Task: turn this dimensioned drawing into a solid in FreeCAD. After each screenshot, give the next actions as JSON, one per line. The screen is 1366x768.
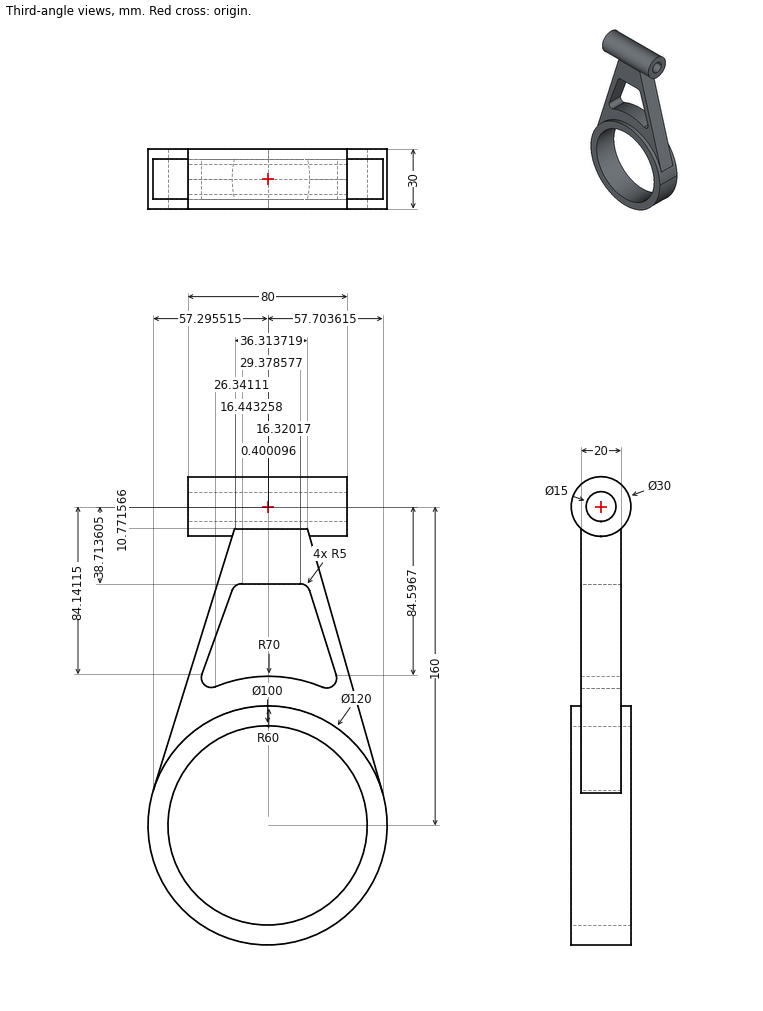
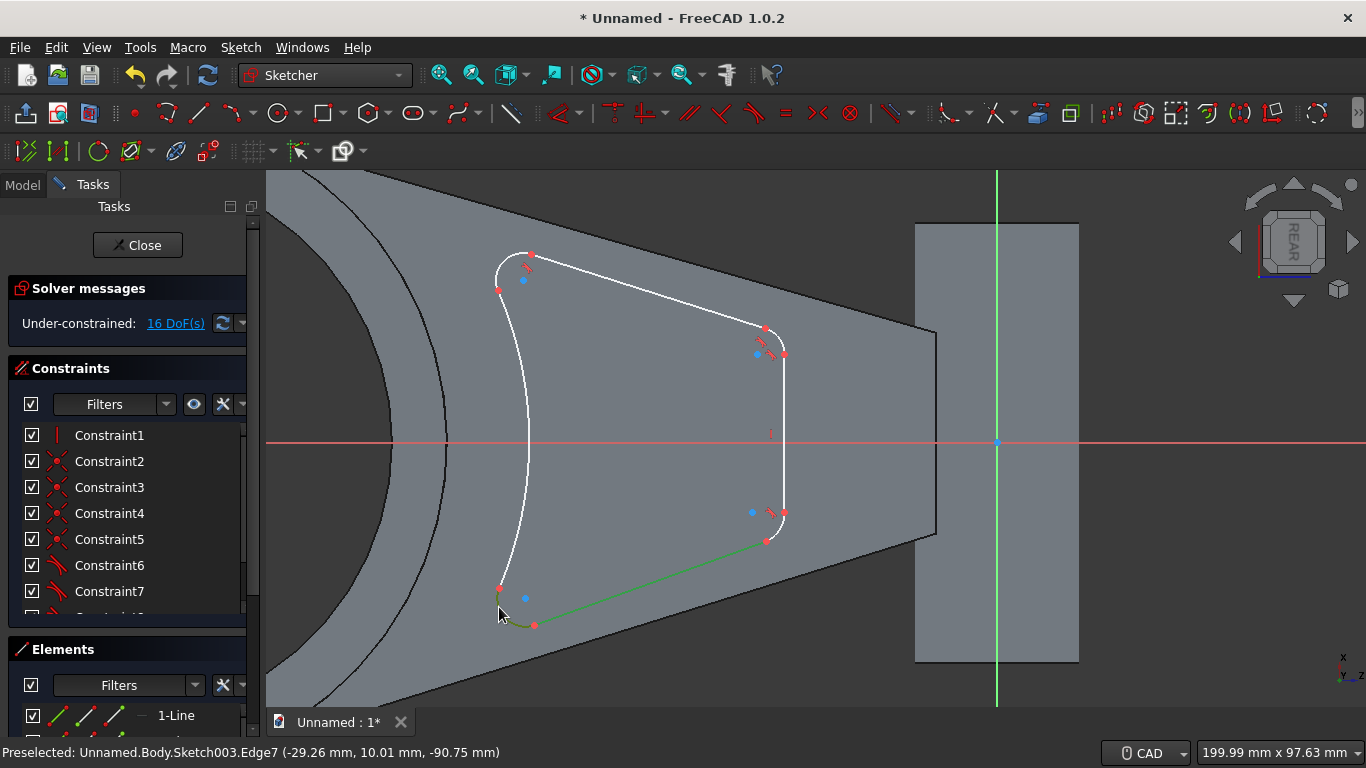
{"action": "left_click", "coordinate": [754, 114]}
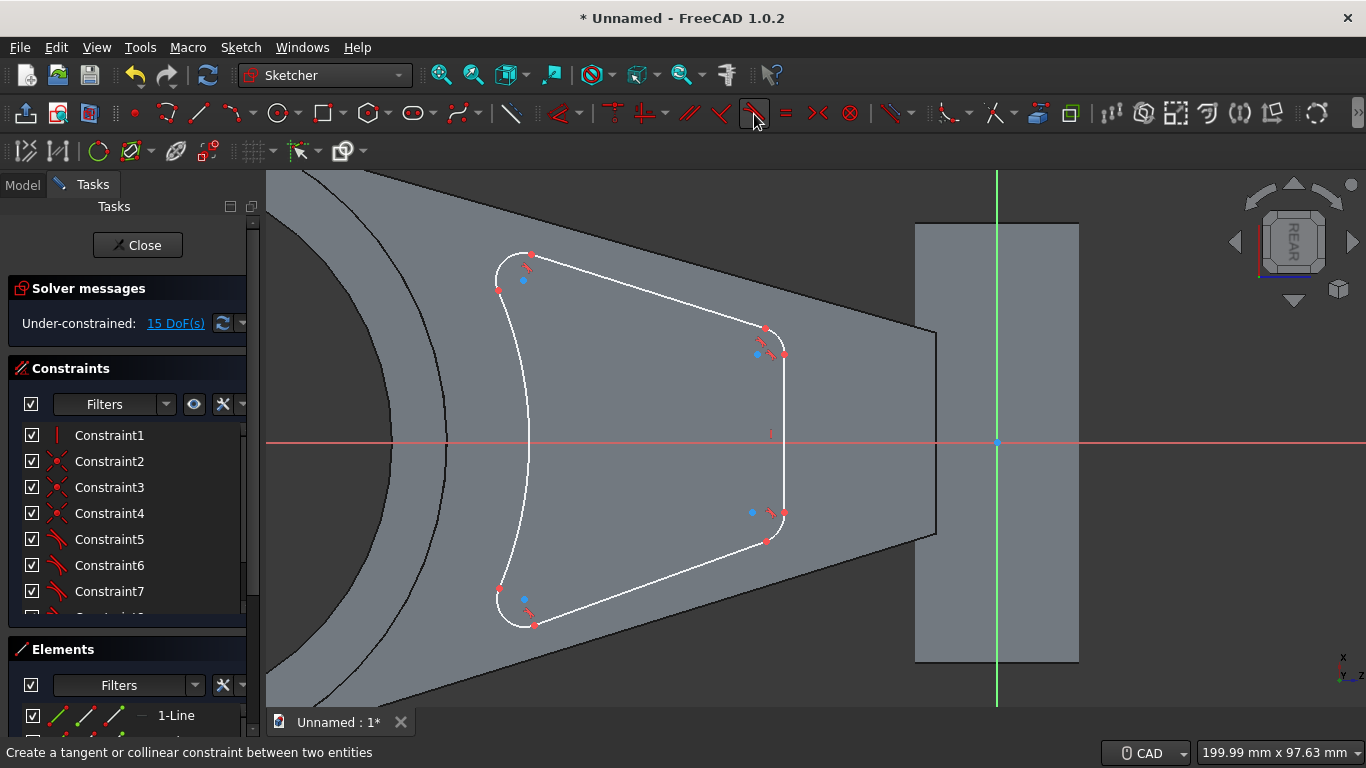
{"action": "left_click", "coordinate": [604, 600]}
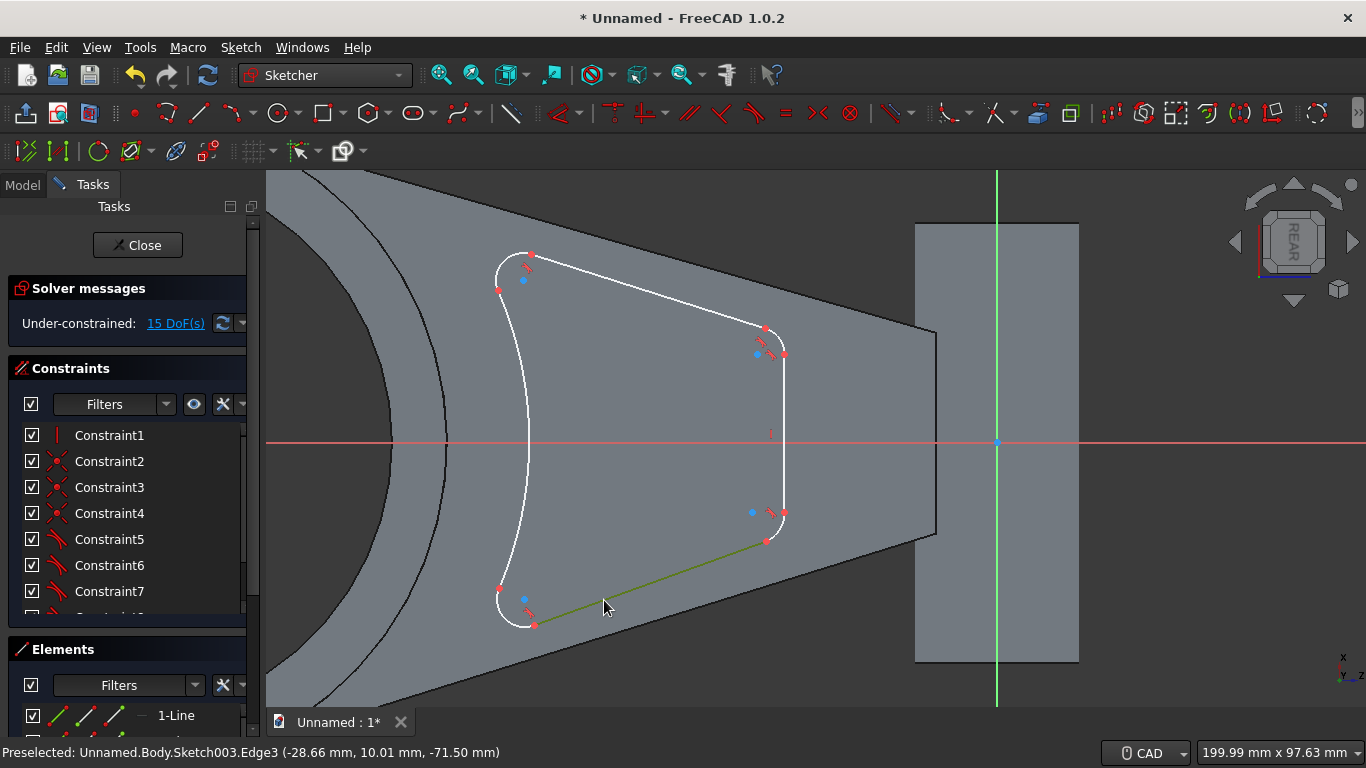
{"action": "scroll", "coordinate": [775, 535], "scroll_direction": "up", "scroll_amount": 2}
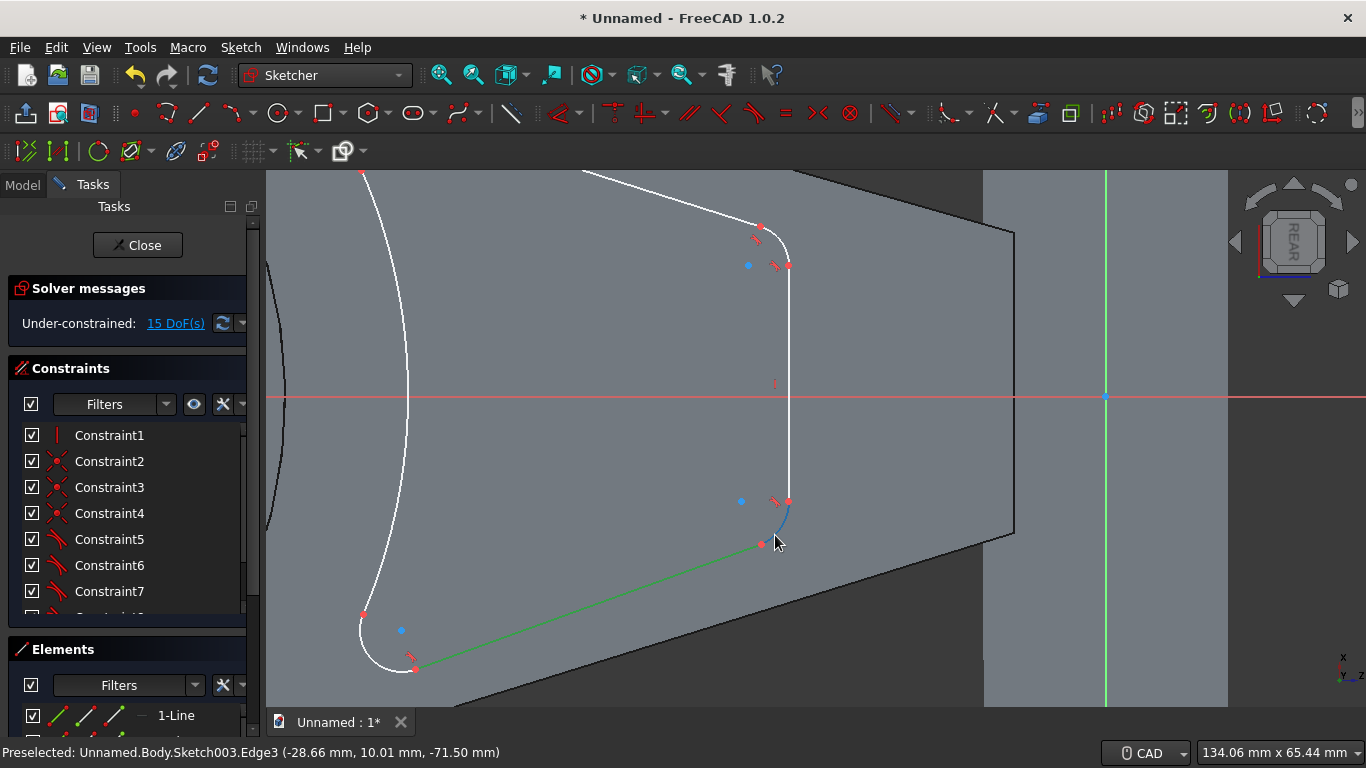
{"action": "left_click", "coordinate": [775, 535]}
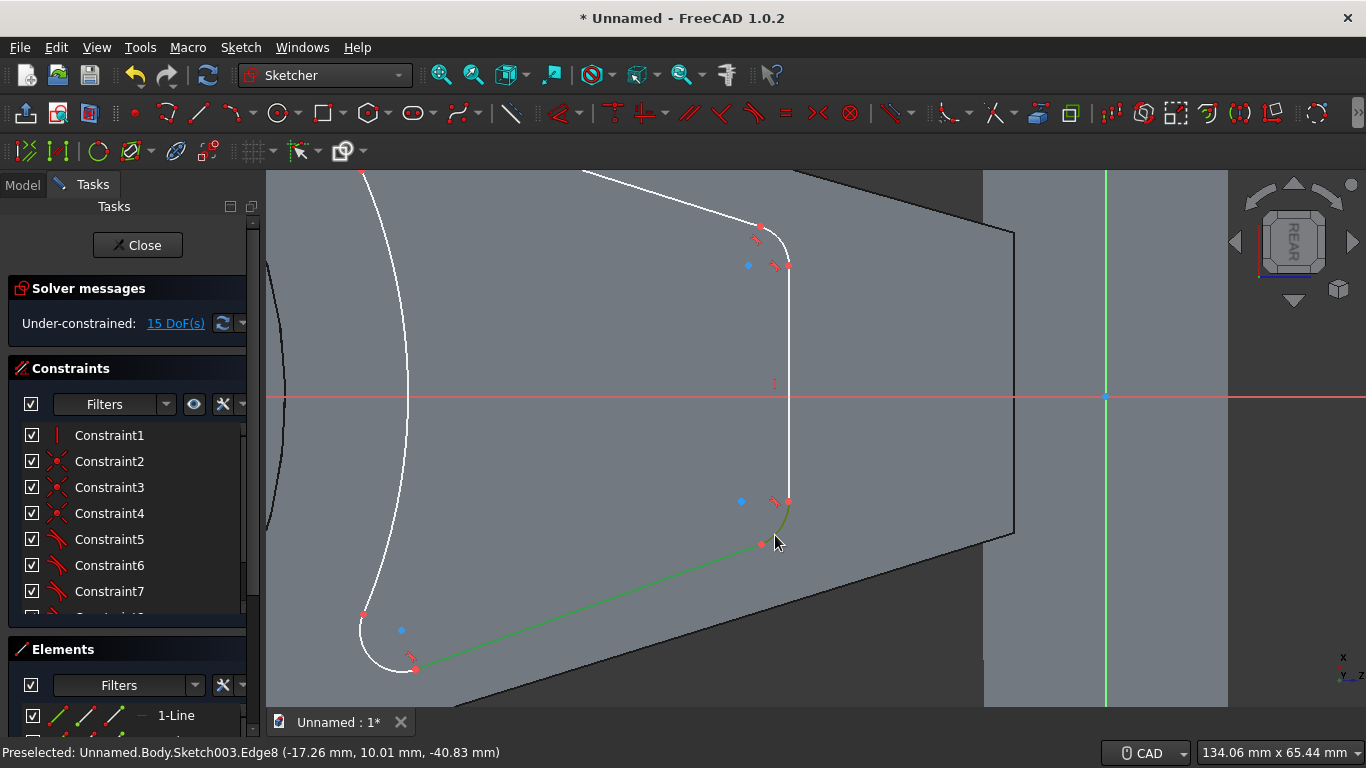
{"action": "left_click", "coordinate": [754, 114]}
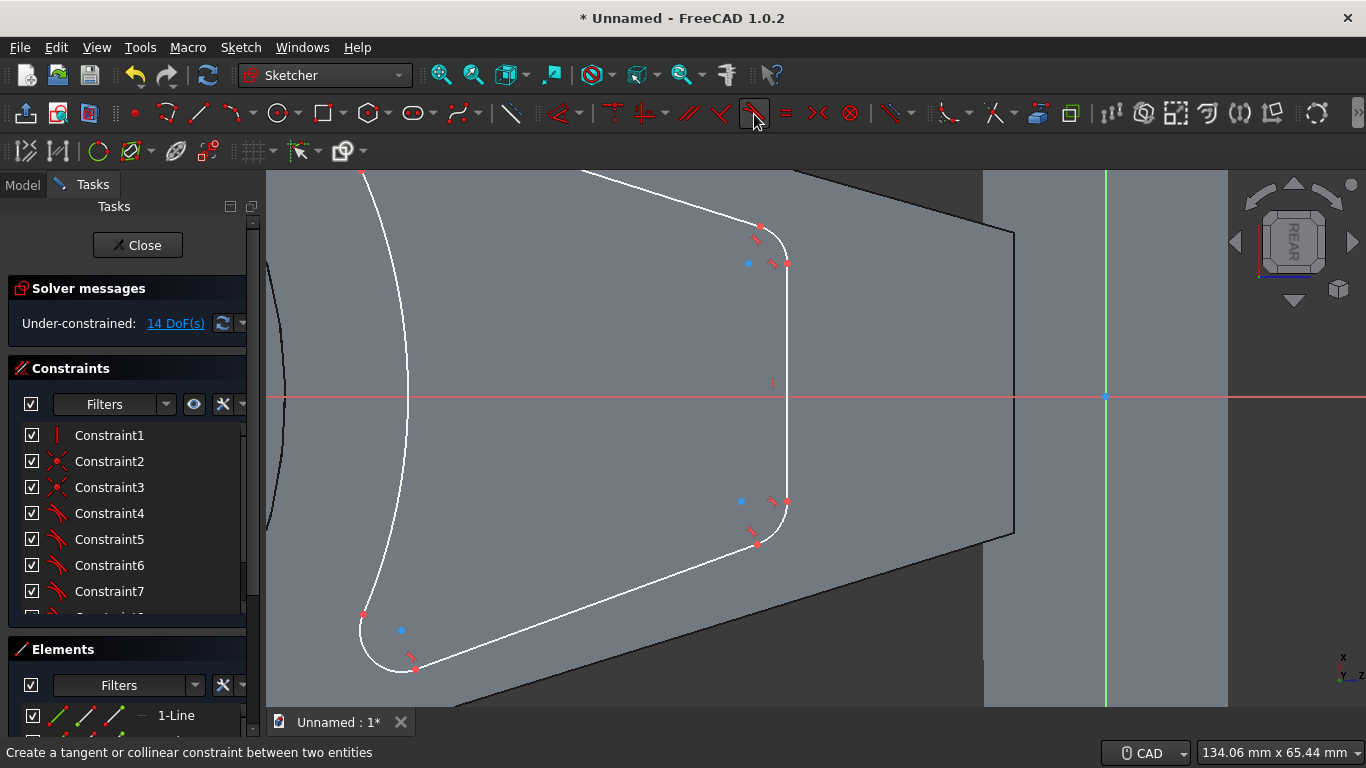
{"action": "scroll", "coordinate": [775, 536], "scroll_direction": "down", "scroll_amount": 2}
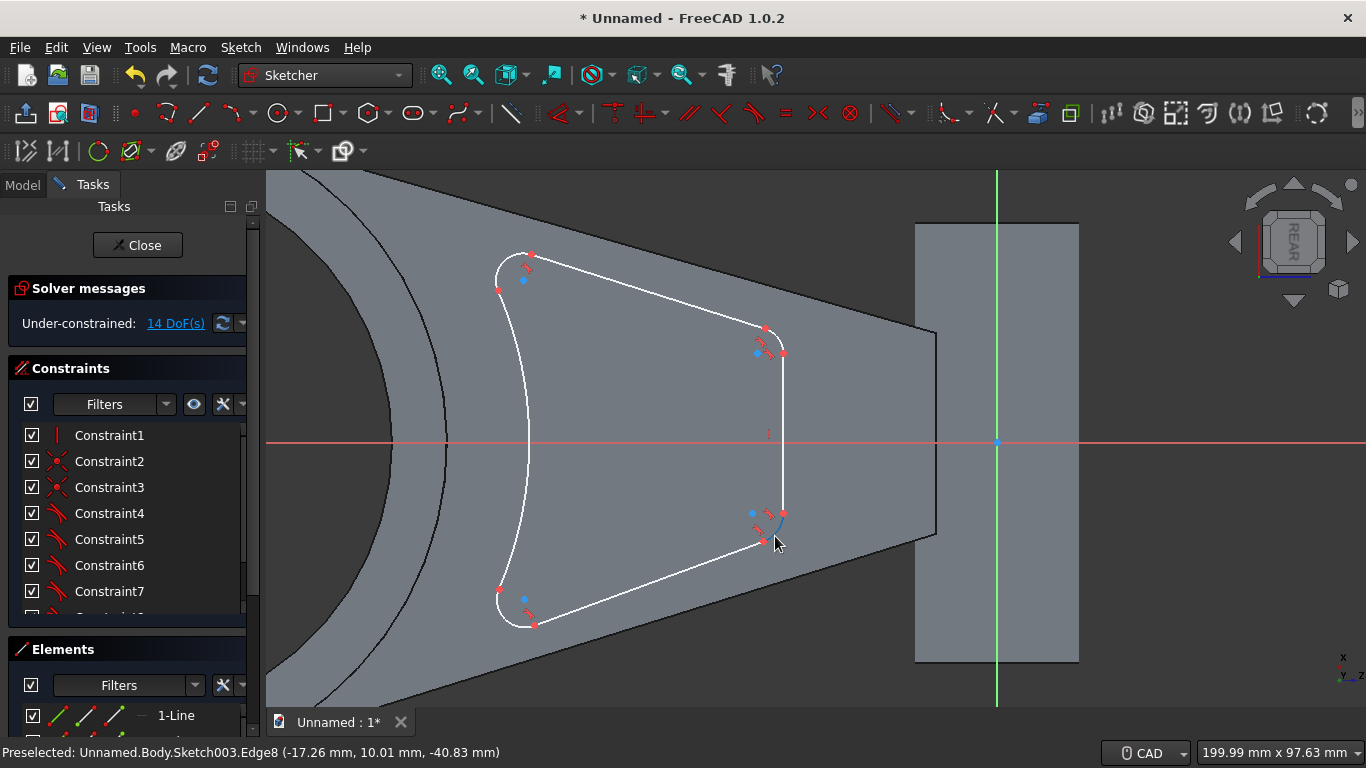
{"action": "left_click", "coordinate": [513, 255]}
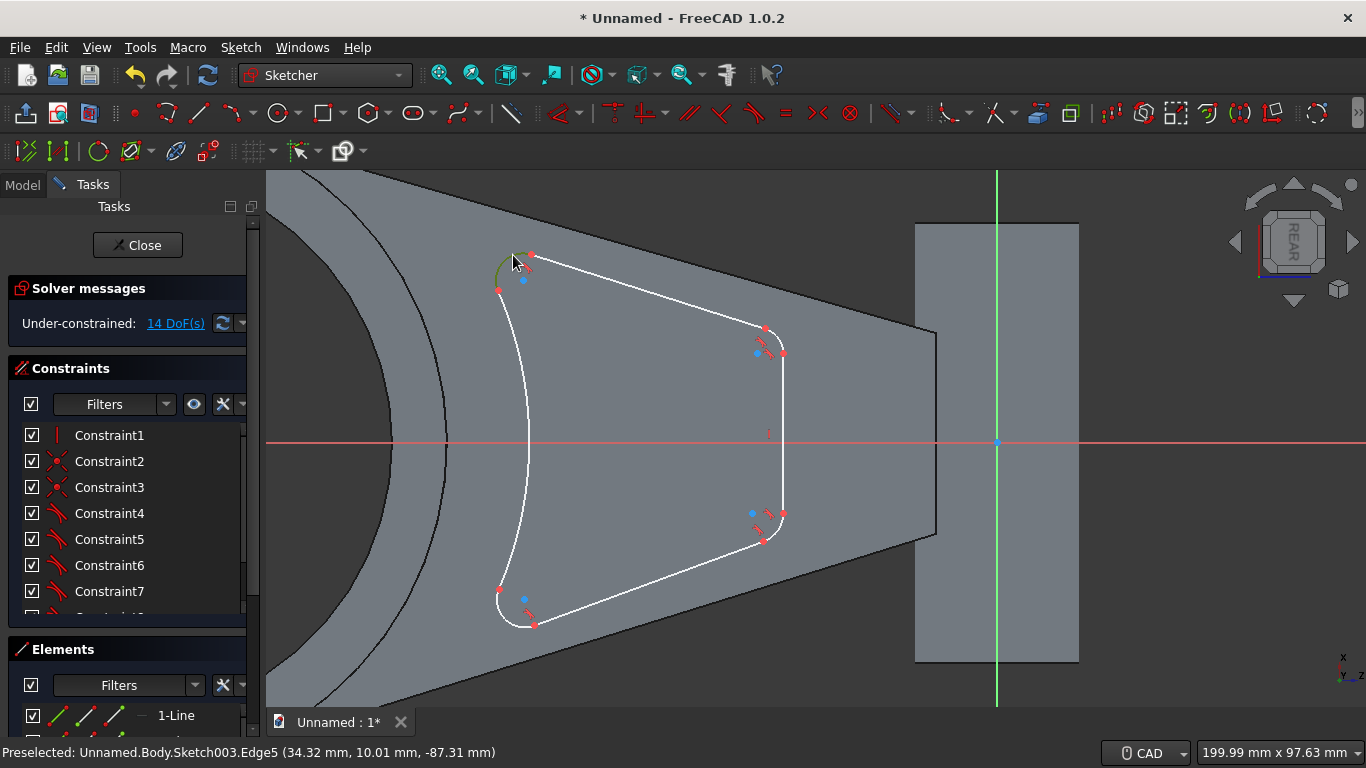
{"action": "left_click", "coordinate": [524, 501]}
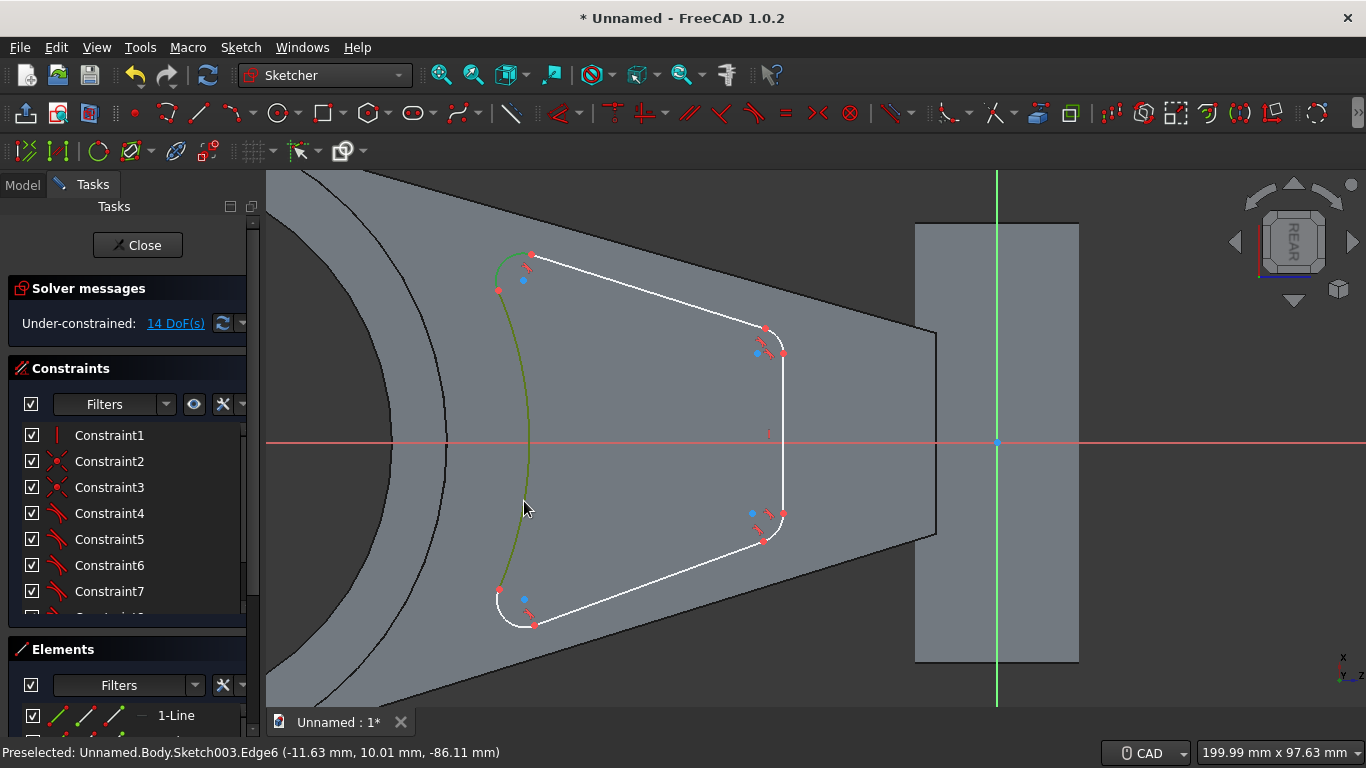
{"action": "key", "text": "t"}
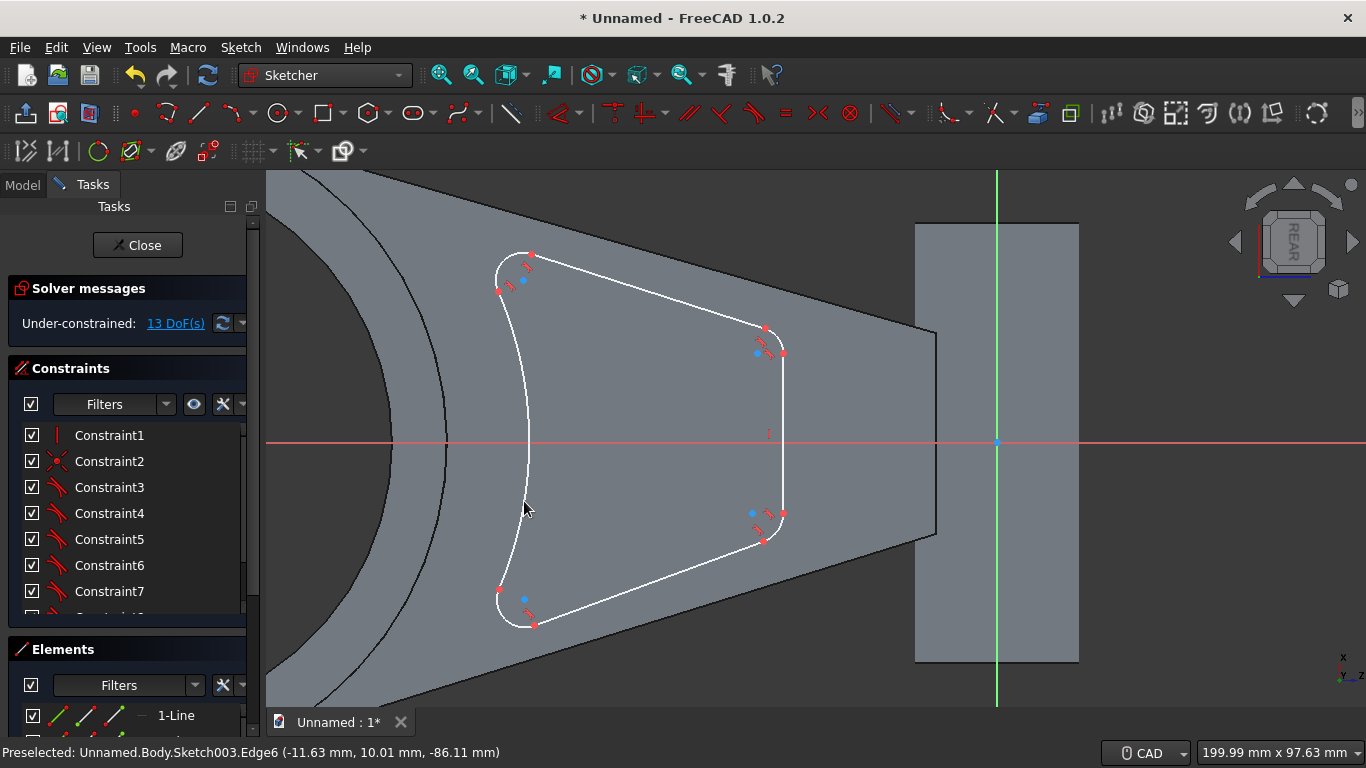
{"action": "left_click", "coordinate": [524, 501]}